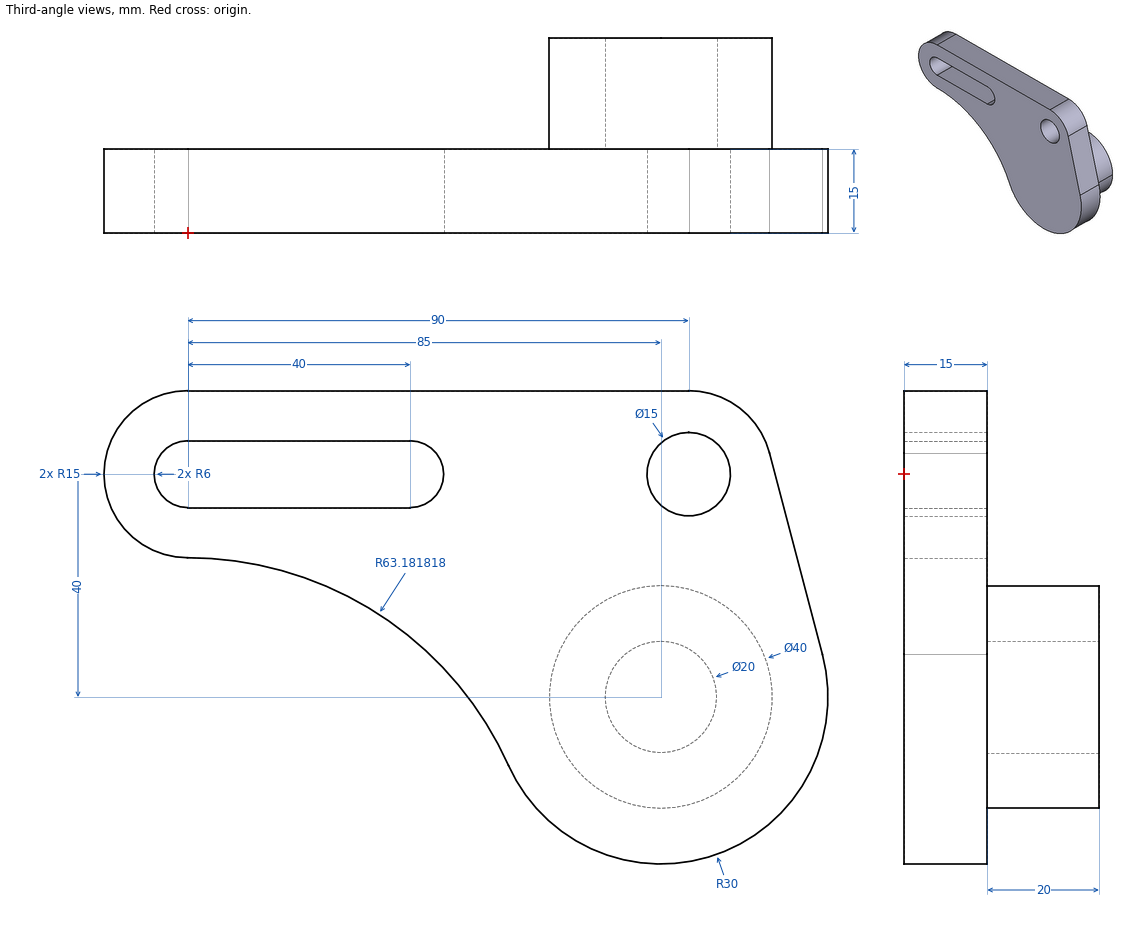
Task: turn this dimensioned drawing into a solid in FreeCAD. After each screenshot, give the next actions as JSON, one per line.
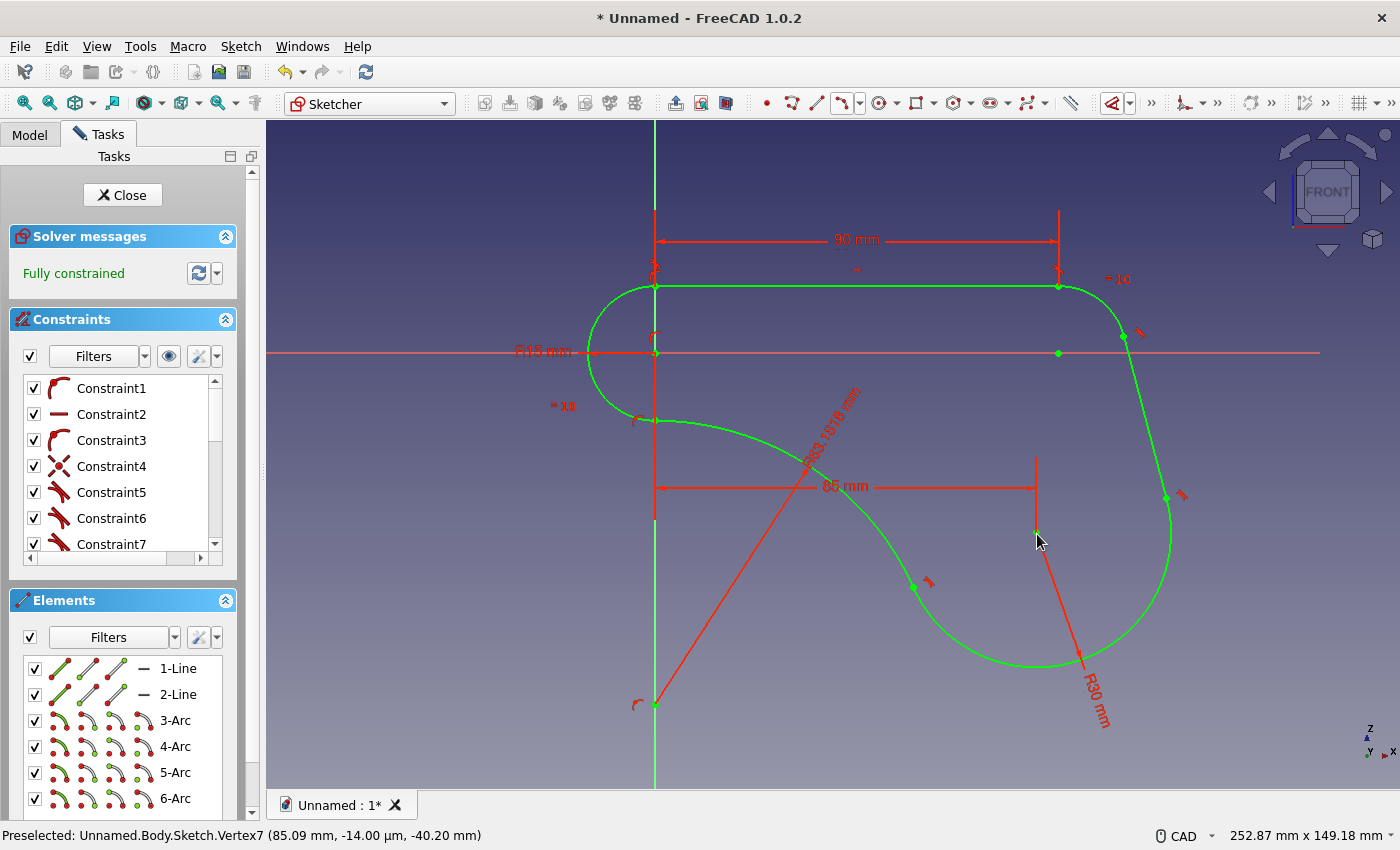
{"action": "left_click", "coordinate": [123, 195]}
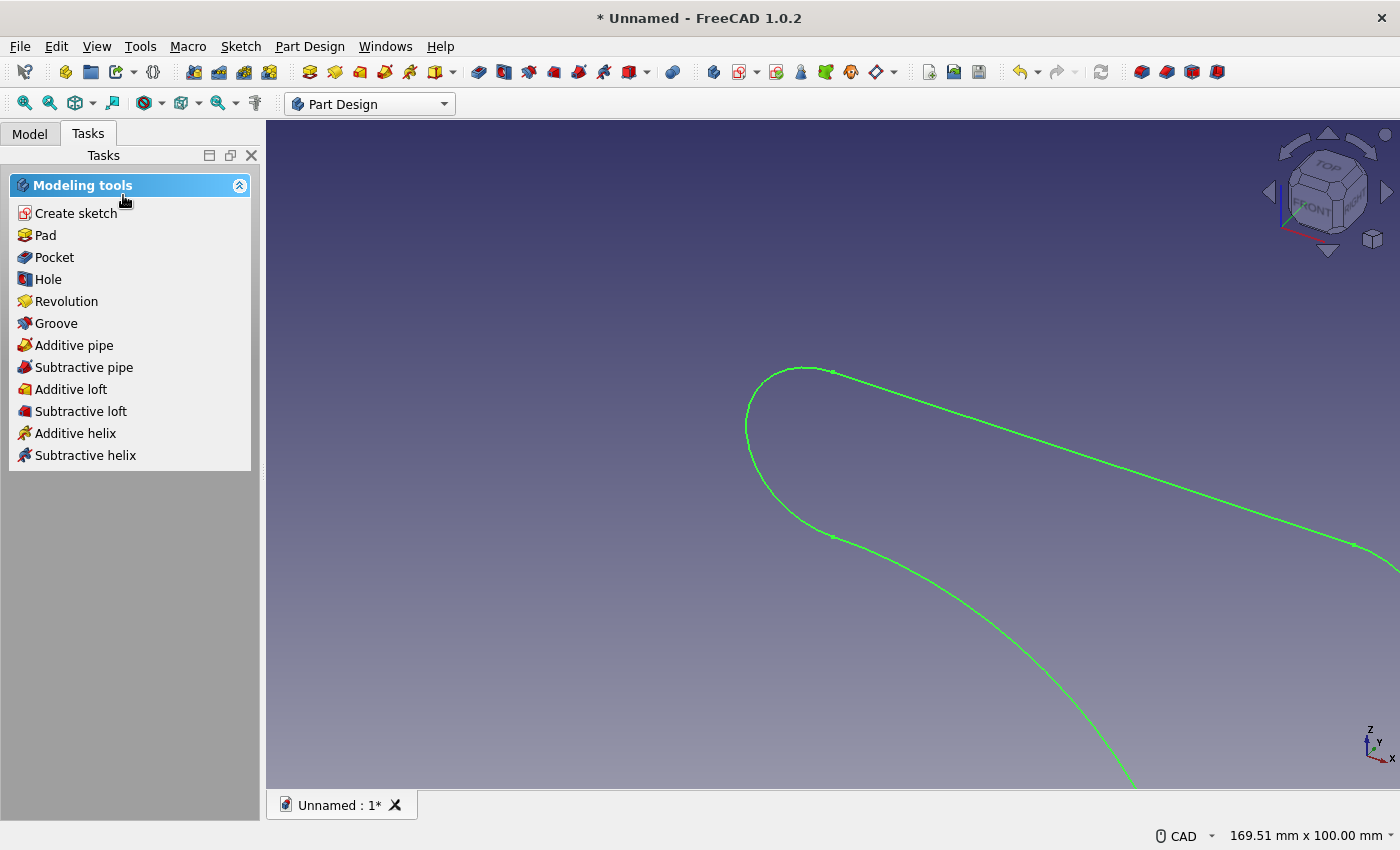
{"action": "left_click", "coordinate": [310, 72]}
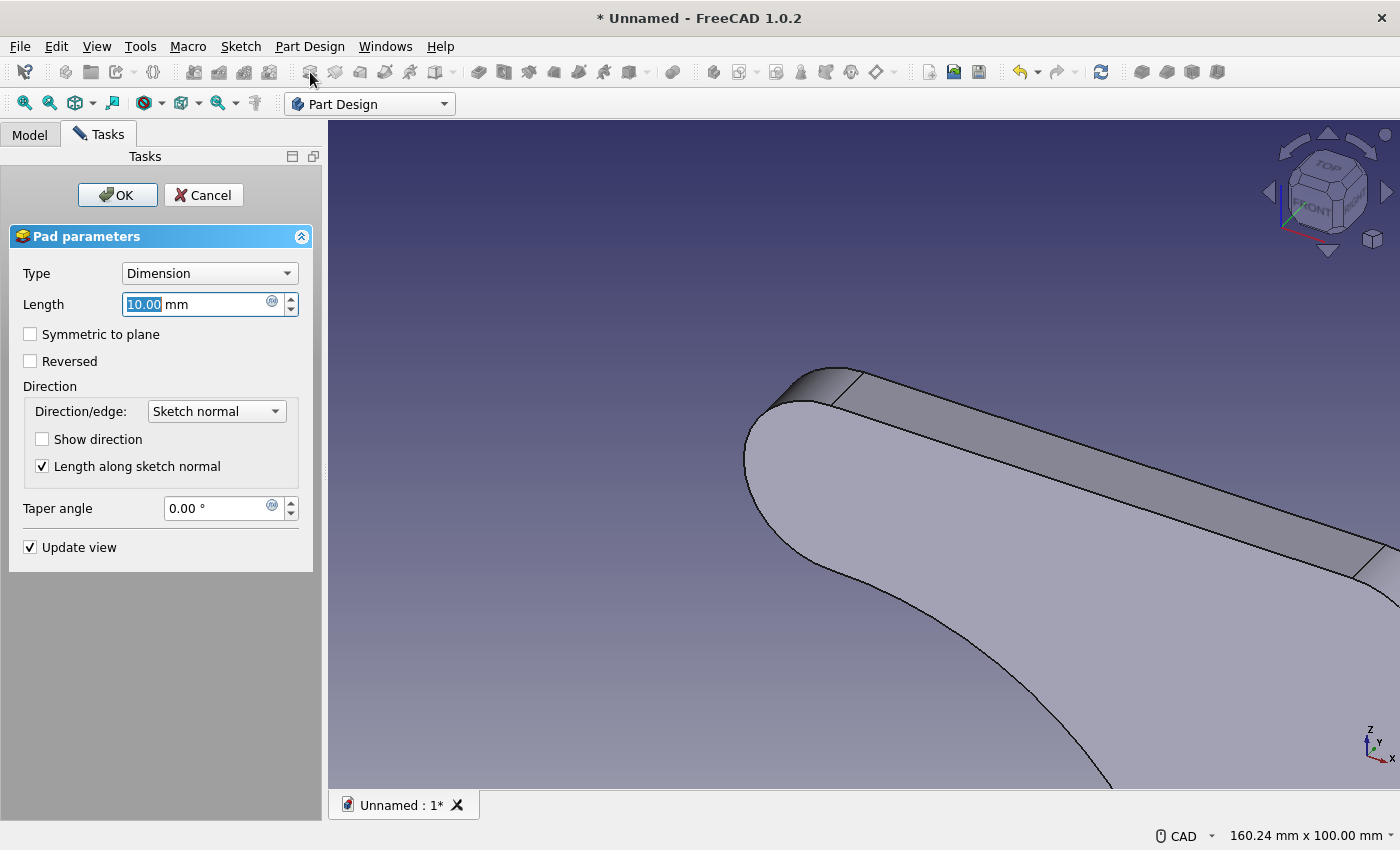
{"action": "type", "text": "15"}
{"action": "key", "text": "Tab"}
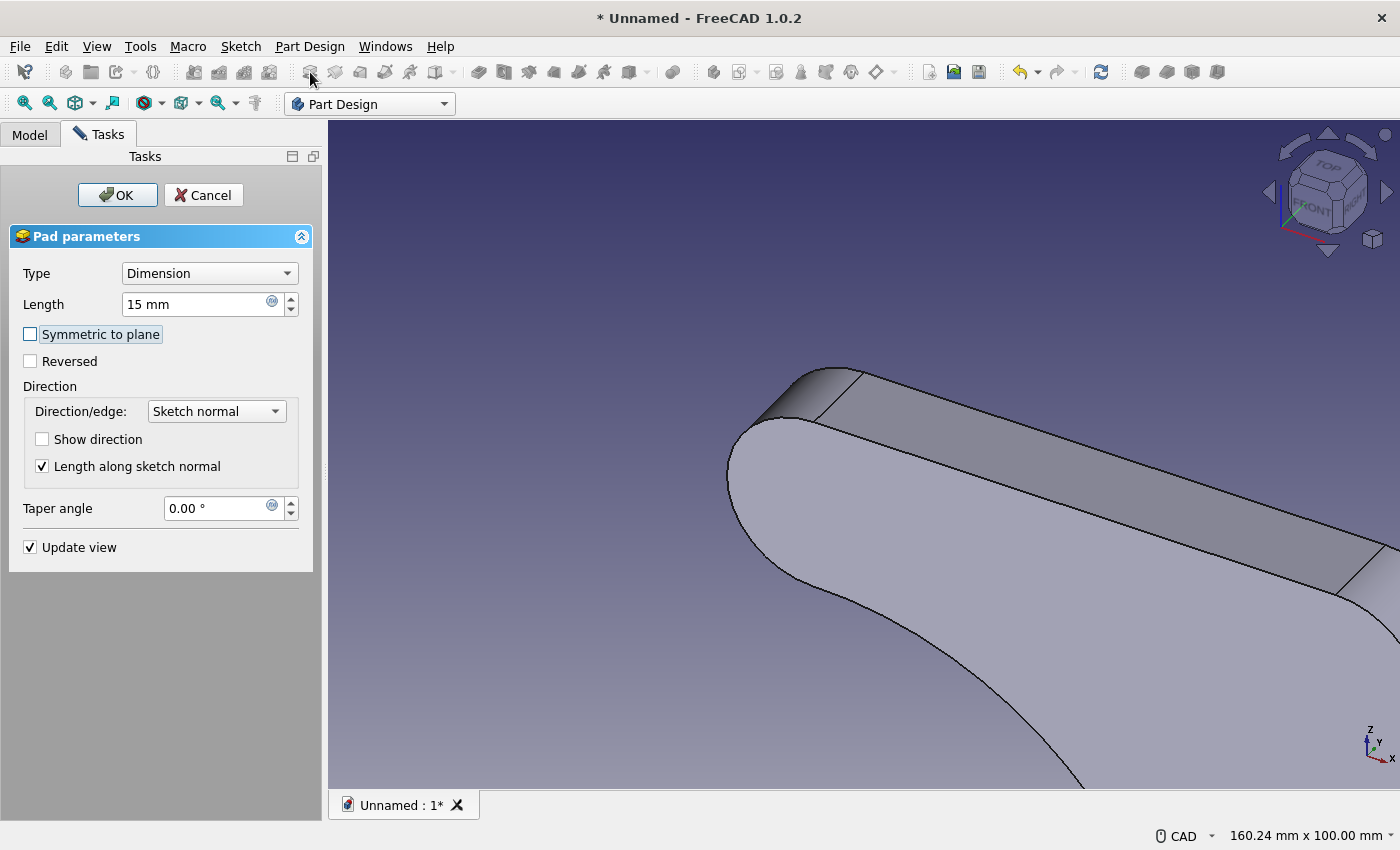
{"action": "left_click", "coordinate": [31, 361]}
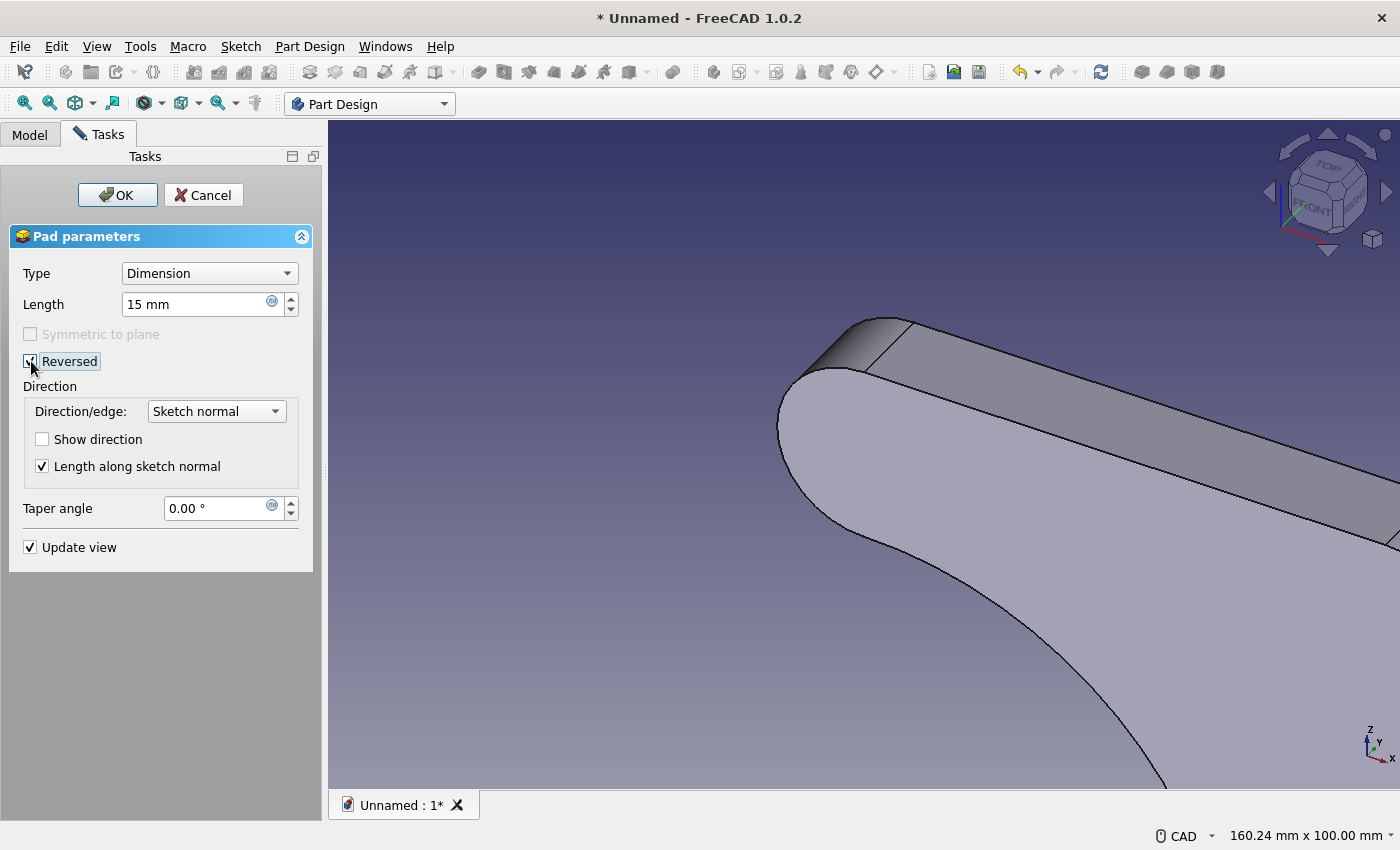
{"action": "left_click", "coordinate": [118, 195]}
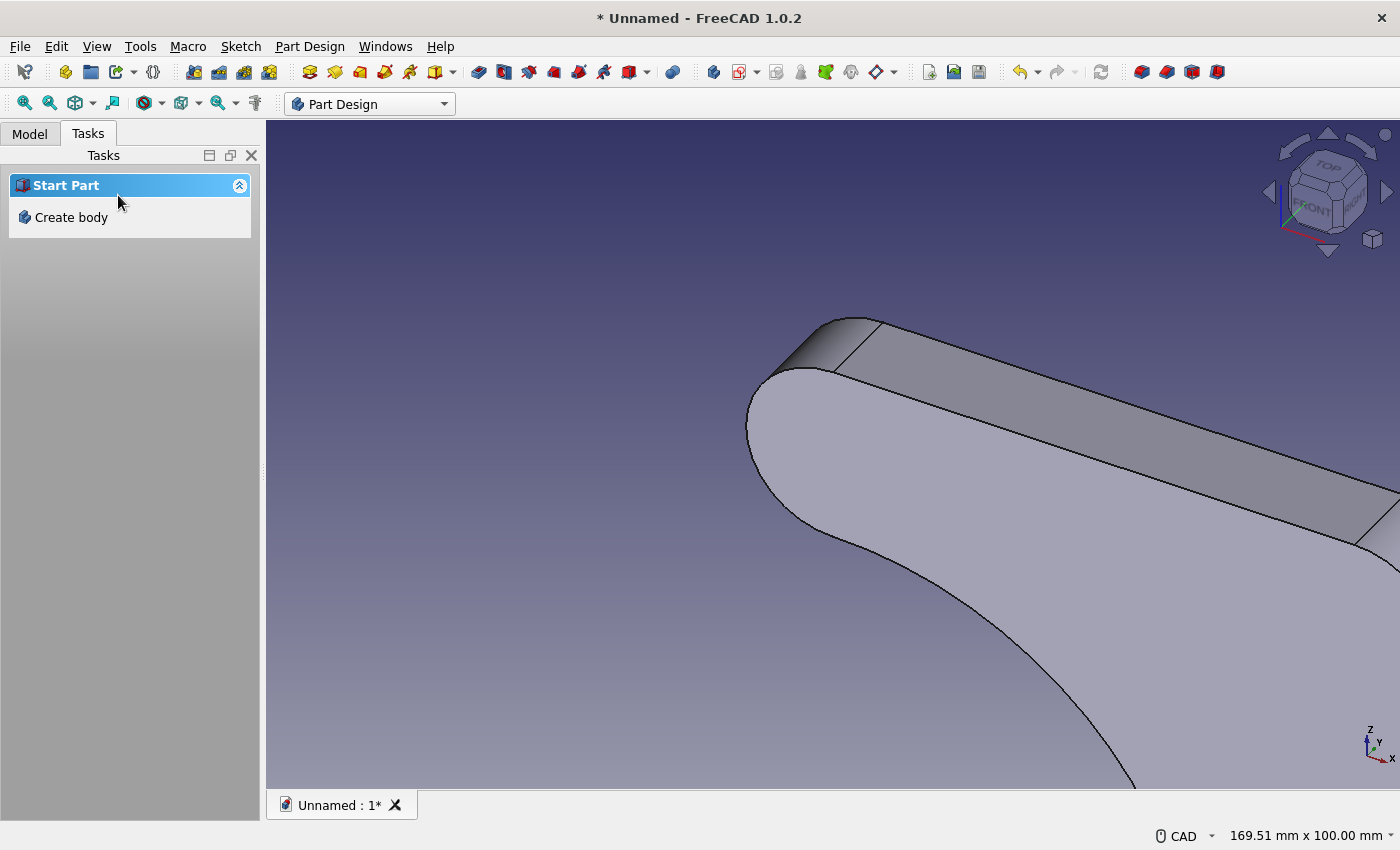
{"action": "left_click", "coordinate": [25, 104]}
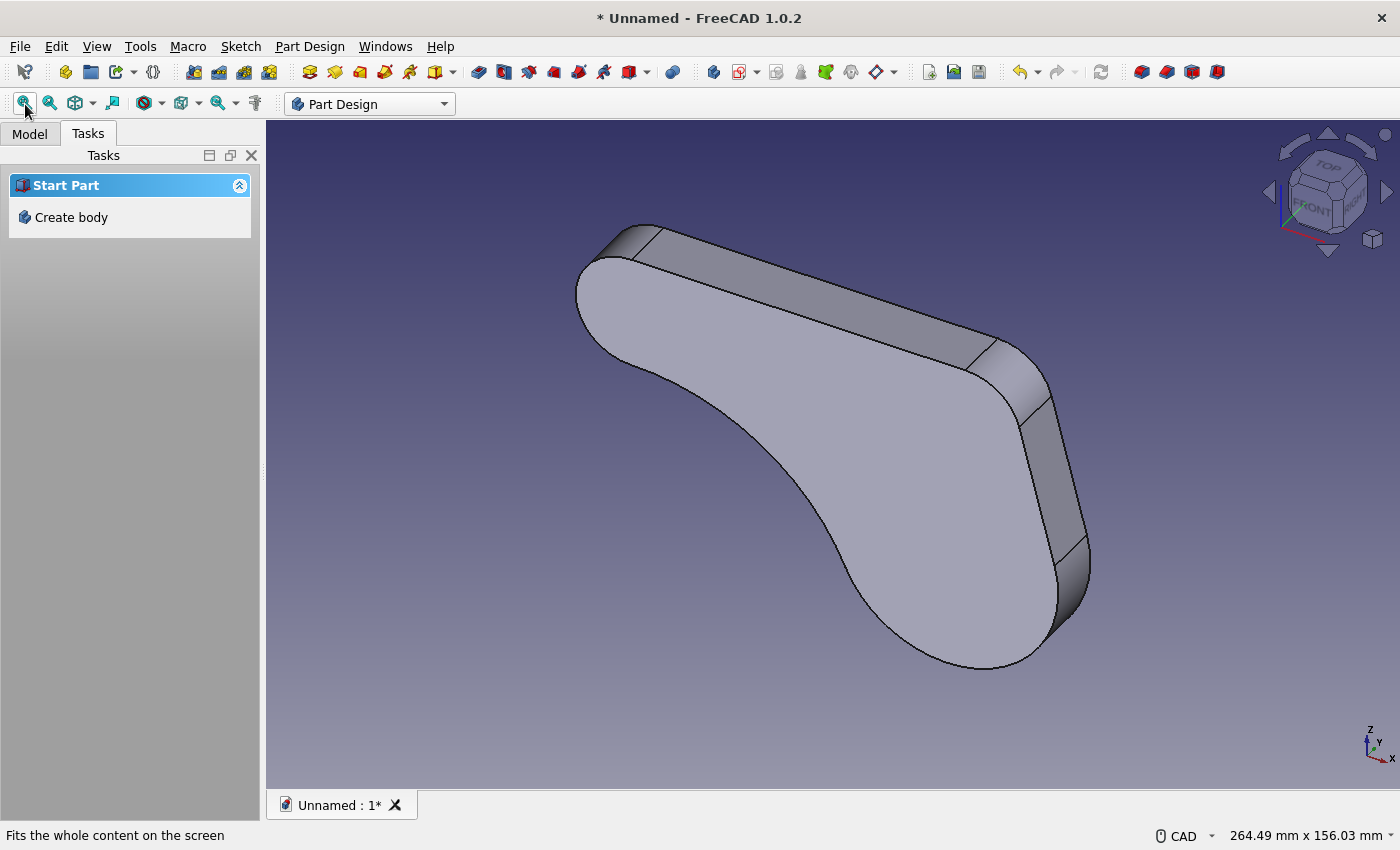
{"action": "key", "text": "4"}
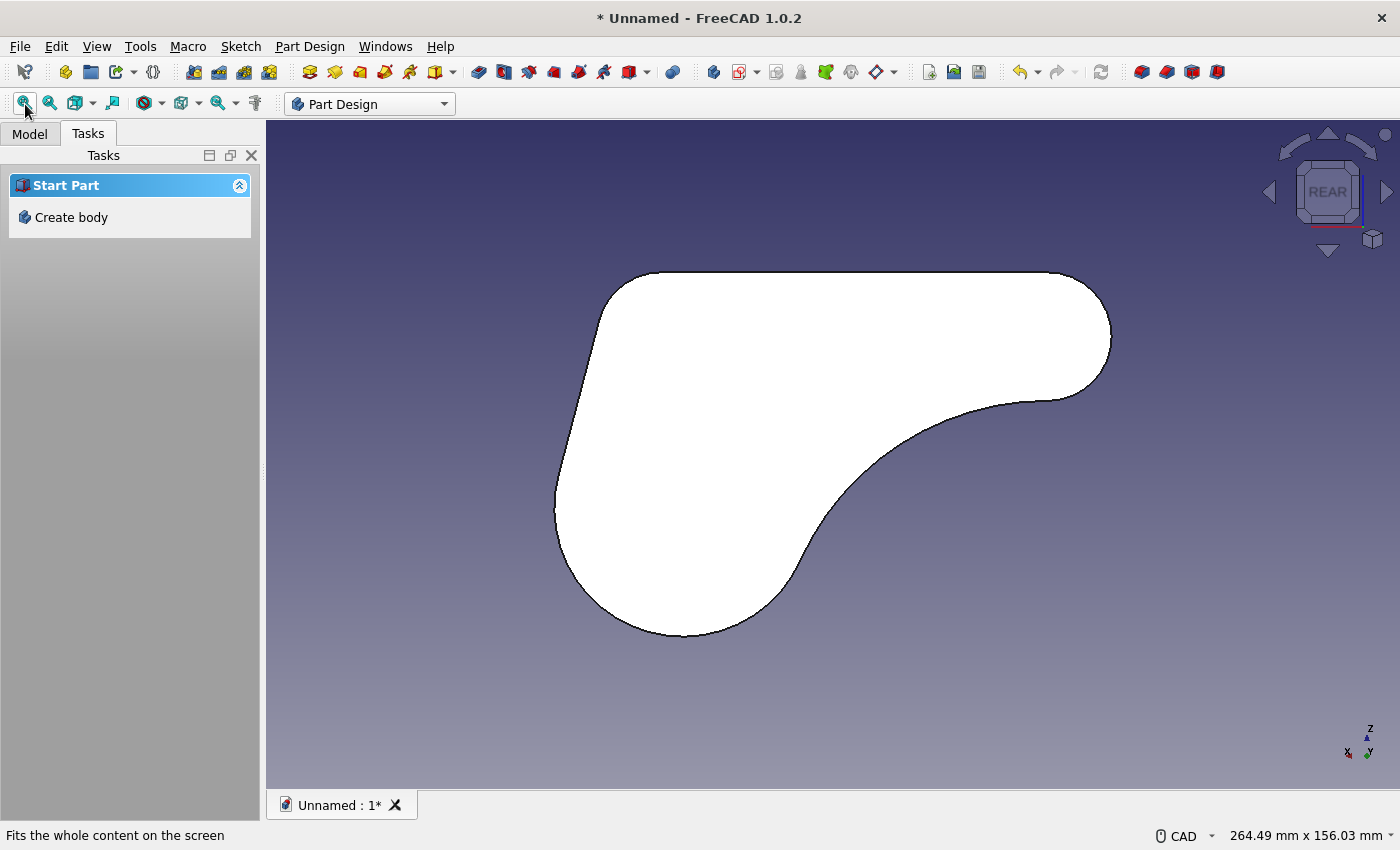
{"action": "left_click", "coordinate": [753, 401]}